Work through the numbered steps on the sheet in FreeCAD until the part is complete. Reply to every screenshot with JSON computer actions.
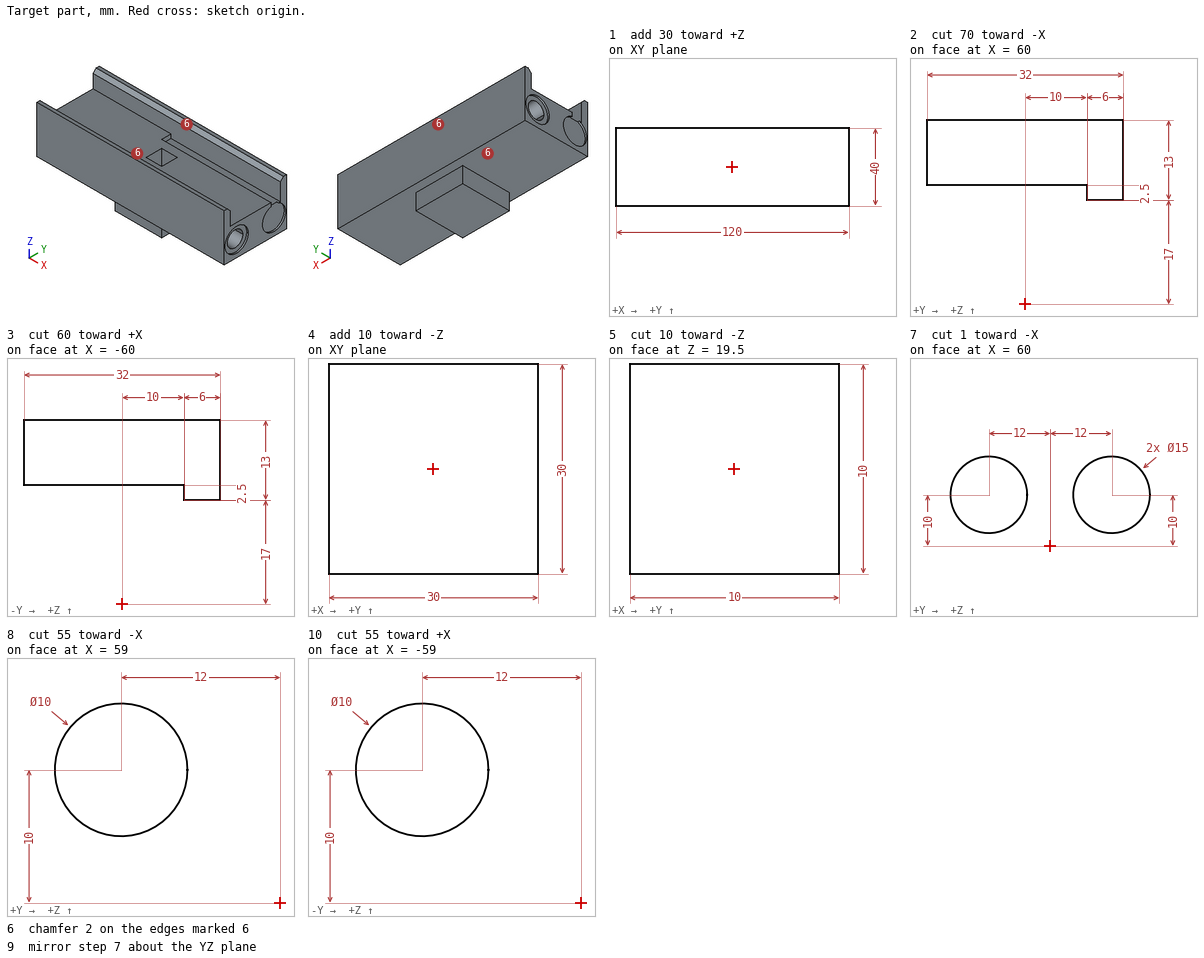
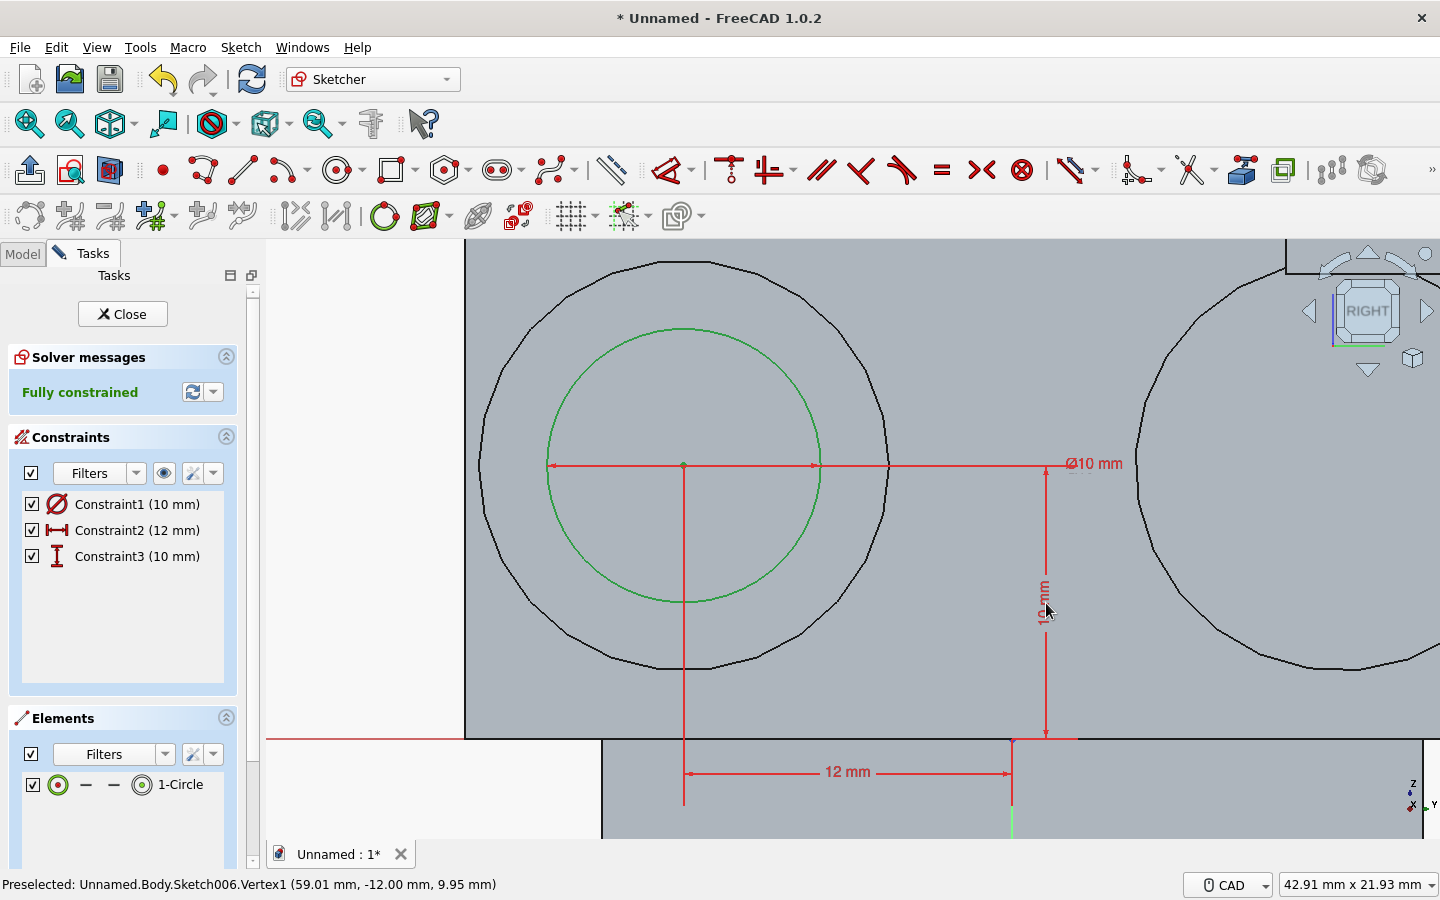
{"action": "left_click", "coordinate": [123, 314]}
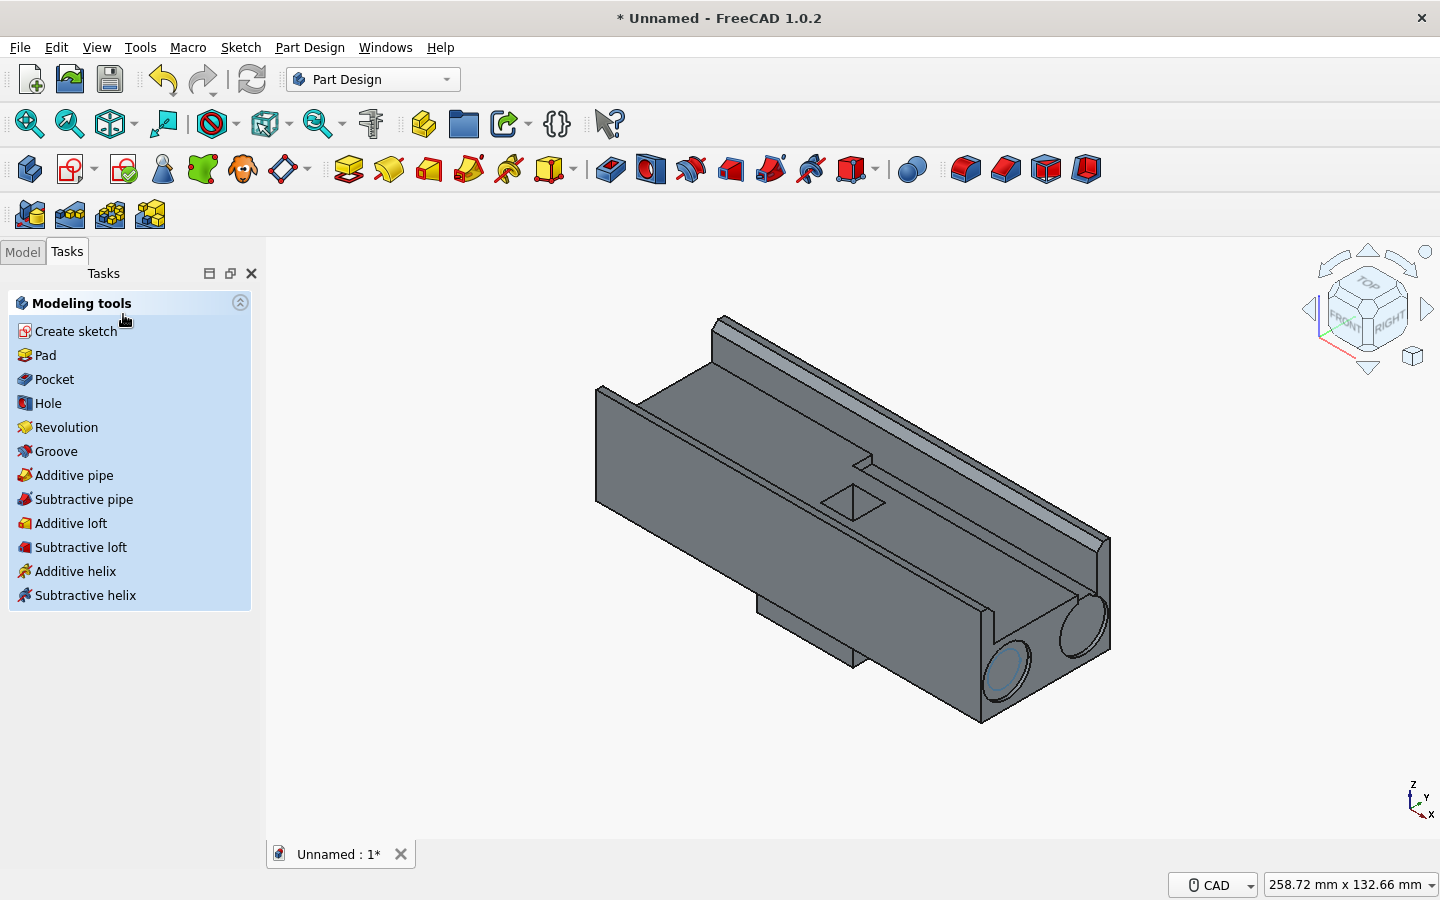
{"action": "left_click", "coordinate": [612, 170]}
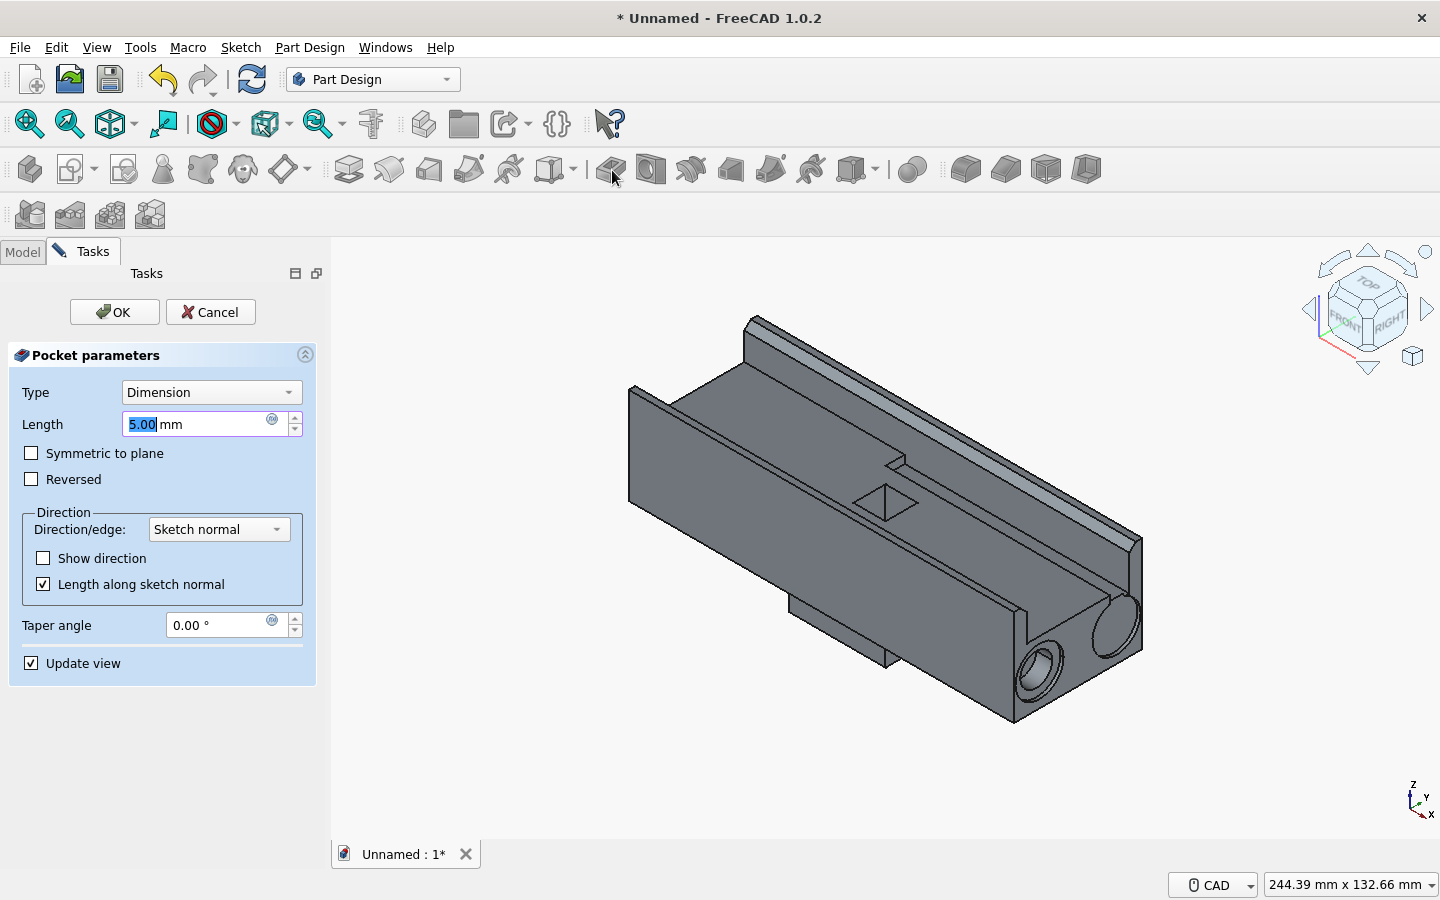
{"action": "type", "text": "55"}
{"action": "key", "text": "Tab"}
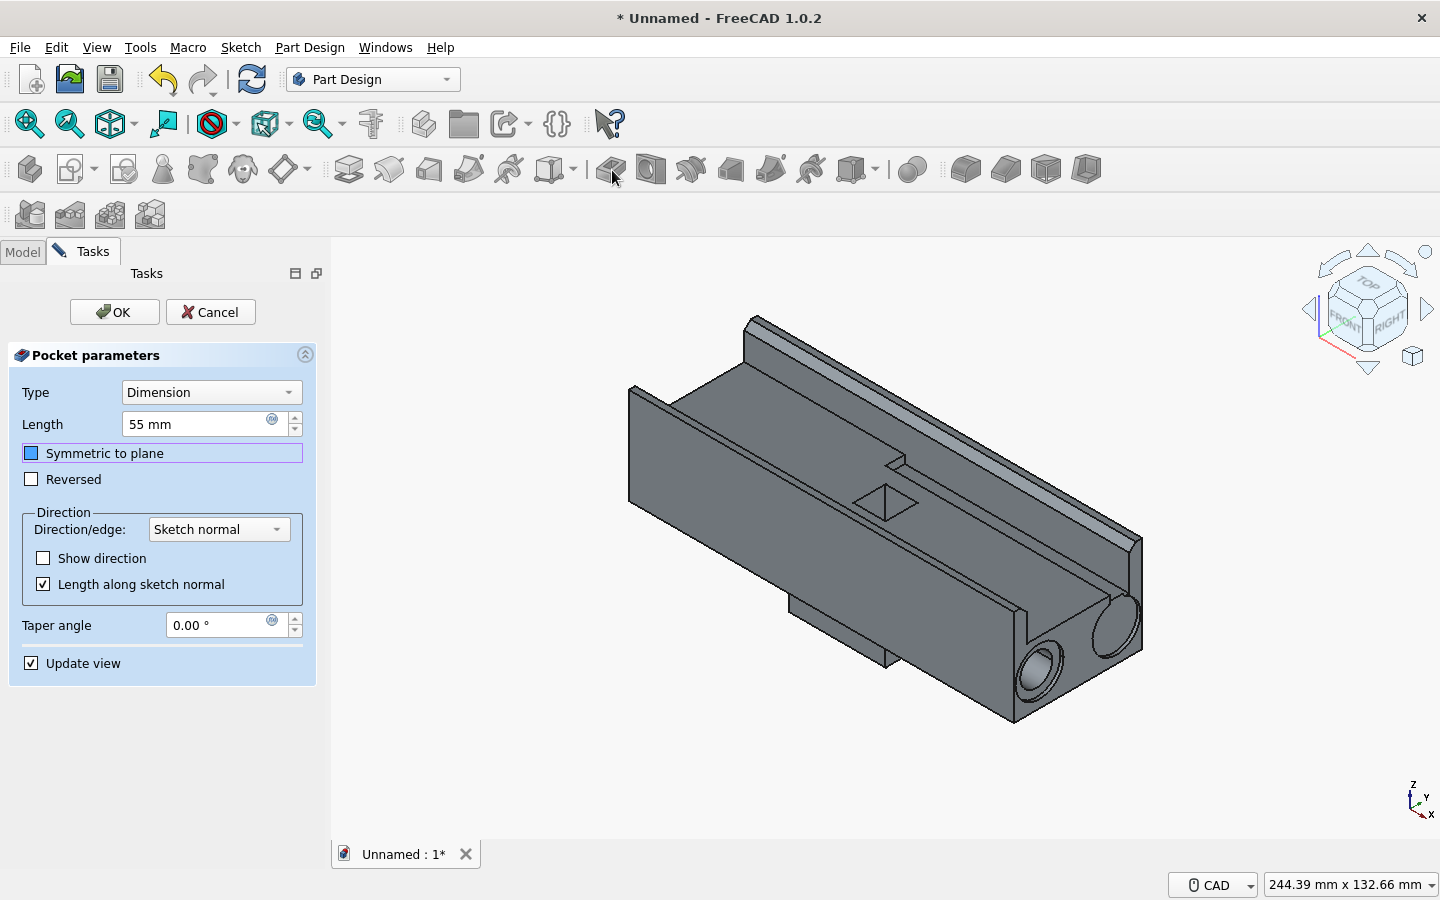
{"action": "left_click", "coordinate": [115, 312]}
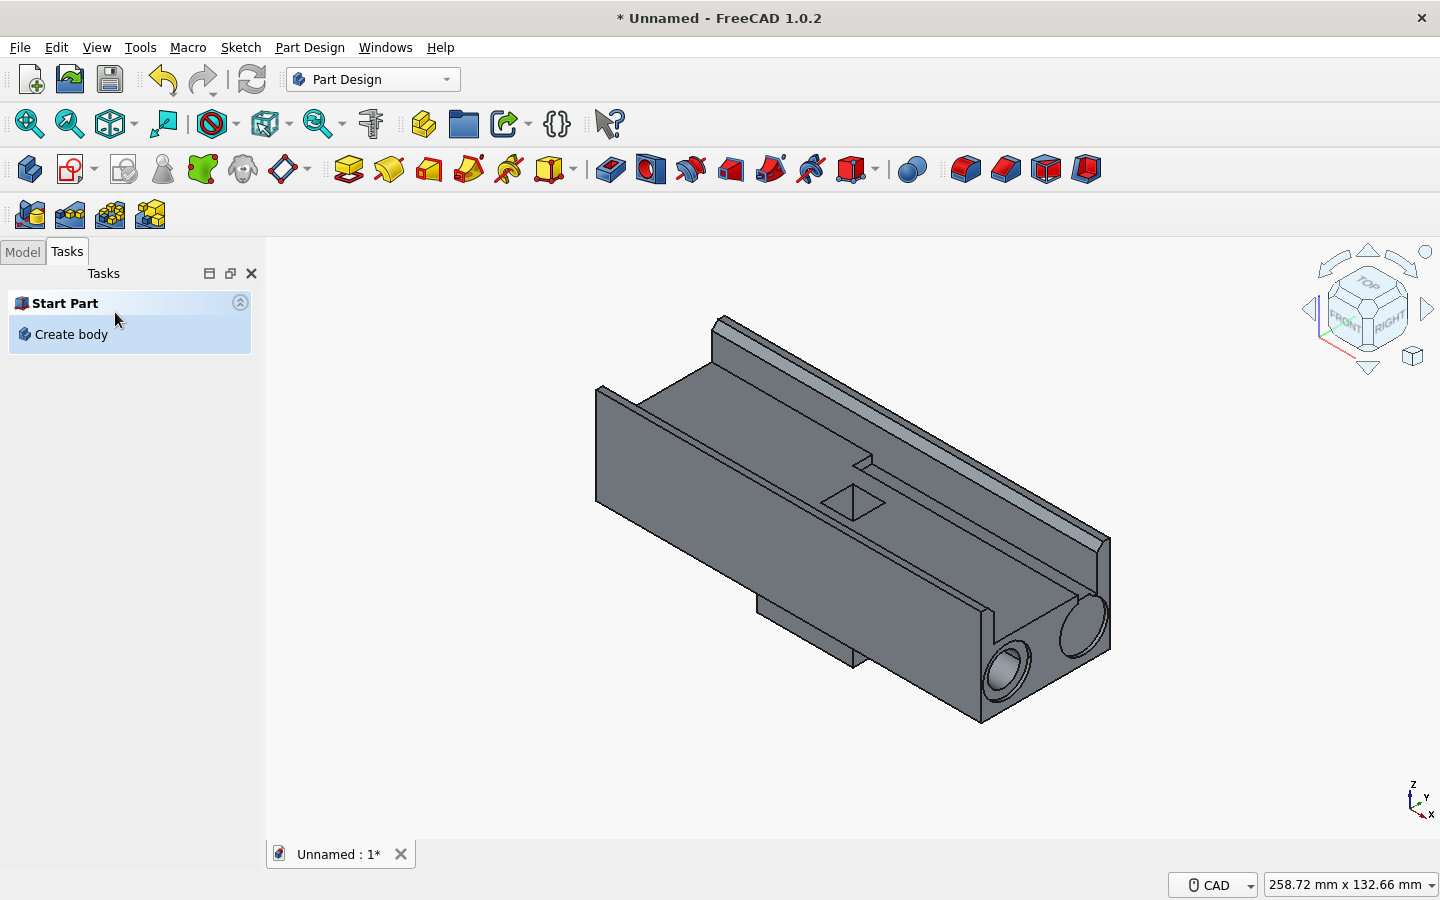
{"action": "left_click", "coordinate": [23, 251]}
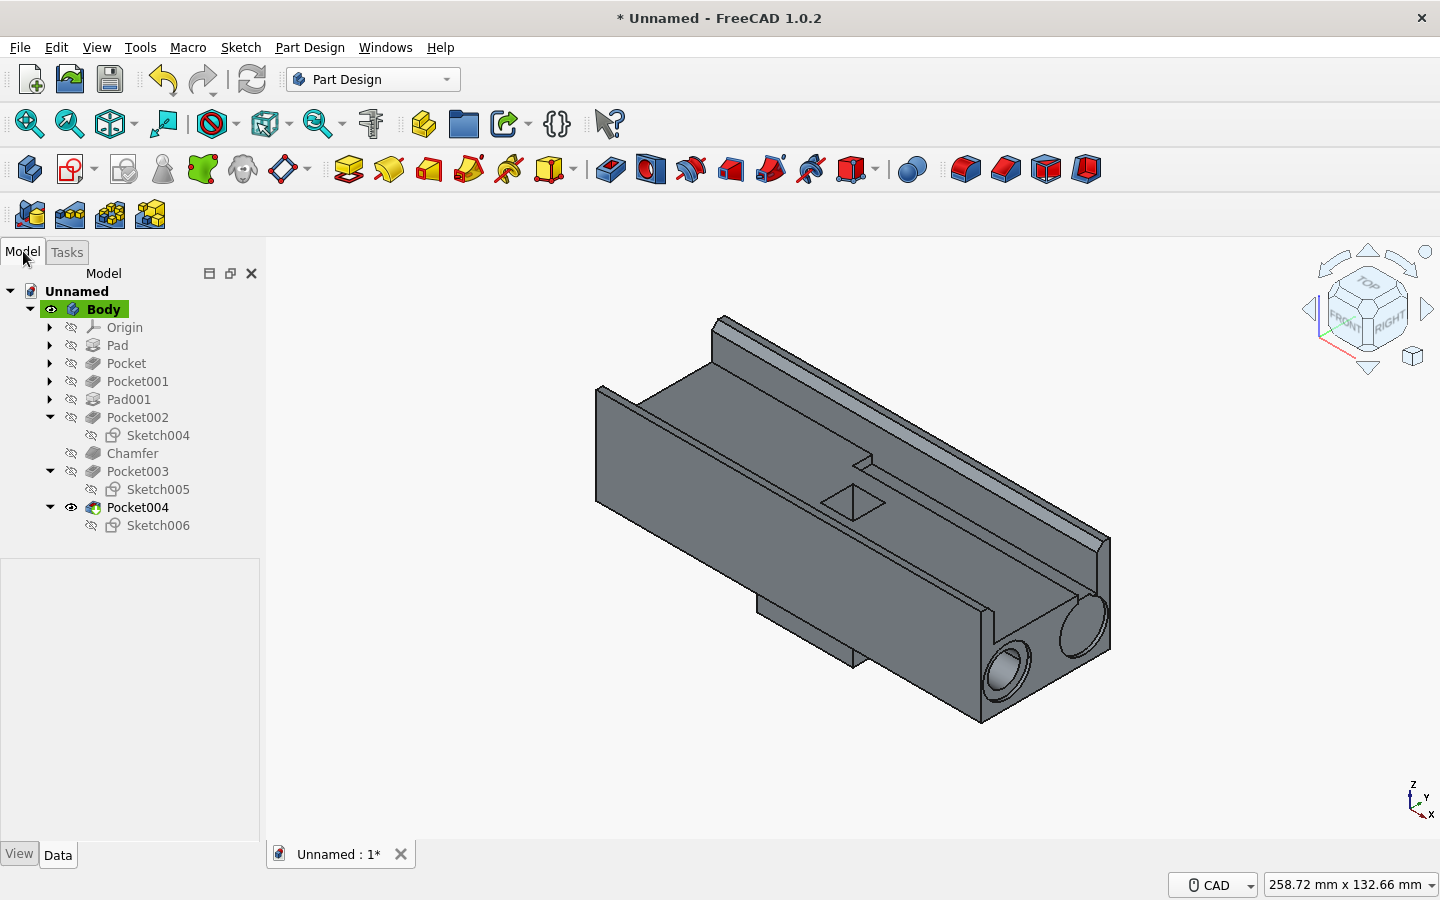
{"action": "left_click", "coordinate": [116, 471]}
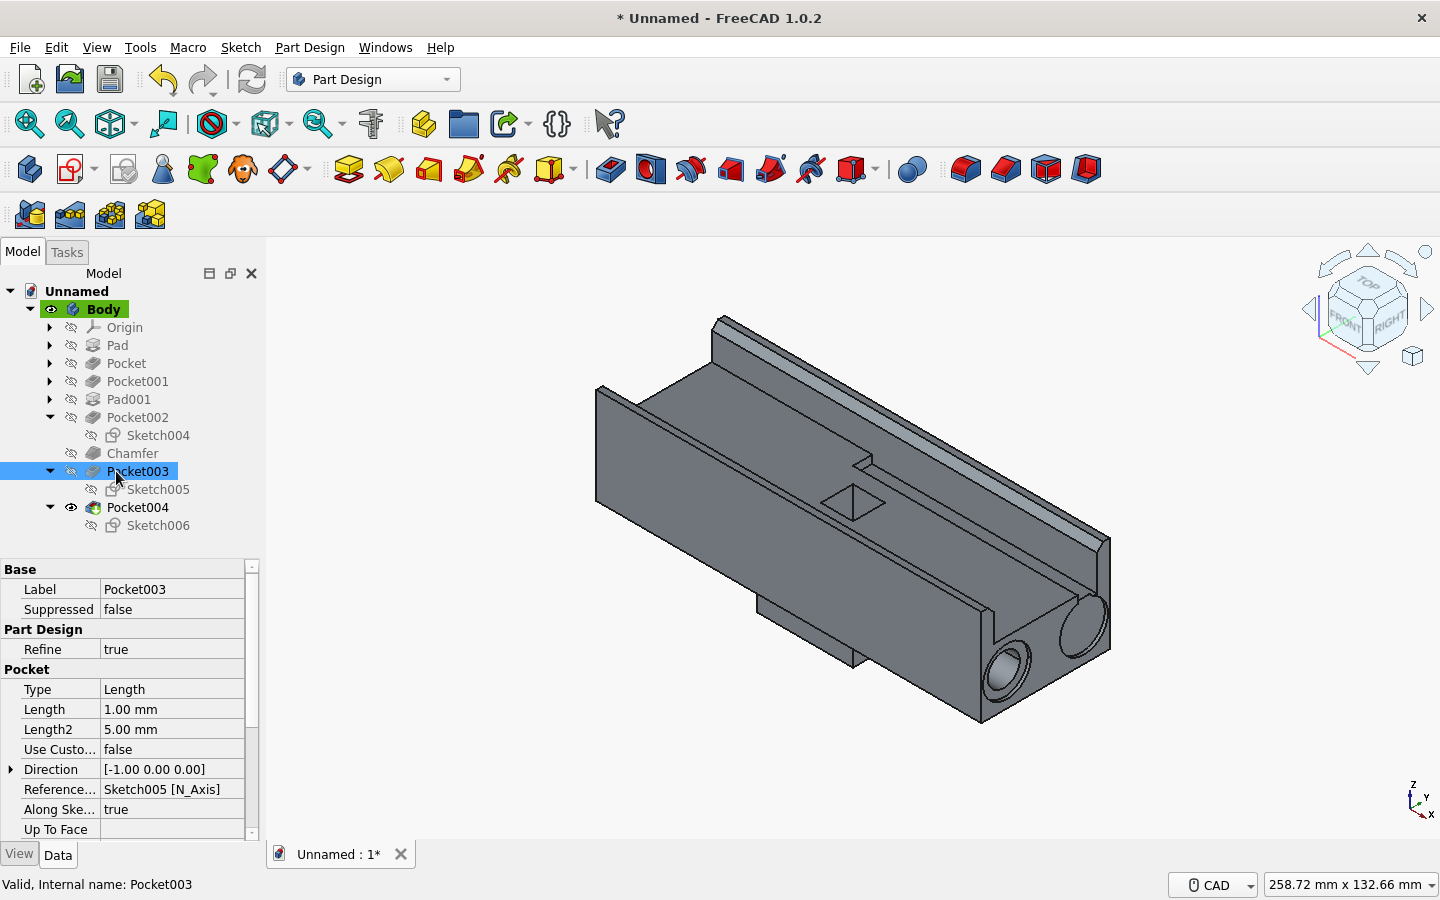
{"action": "left_click", "coordinate": [30, 214]}